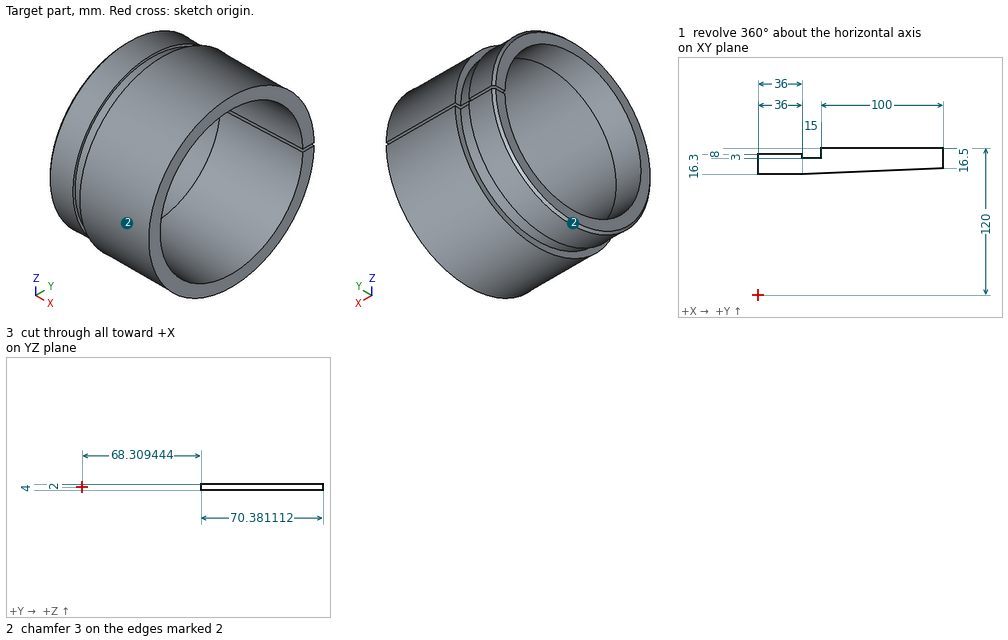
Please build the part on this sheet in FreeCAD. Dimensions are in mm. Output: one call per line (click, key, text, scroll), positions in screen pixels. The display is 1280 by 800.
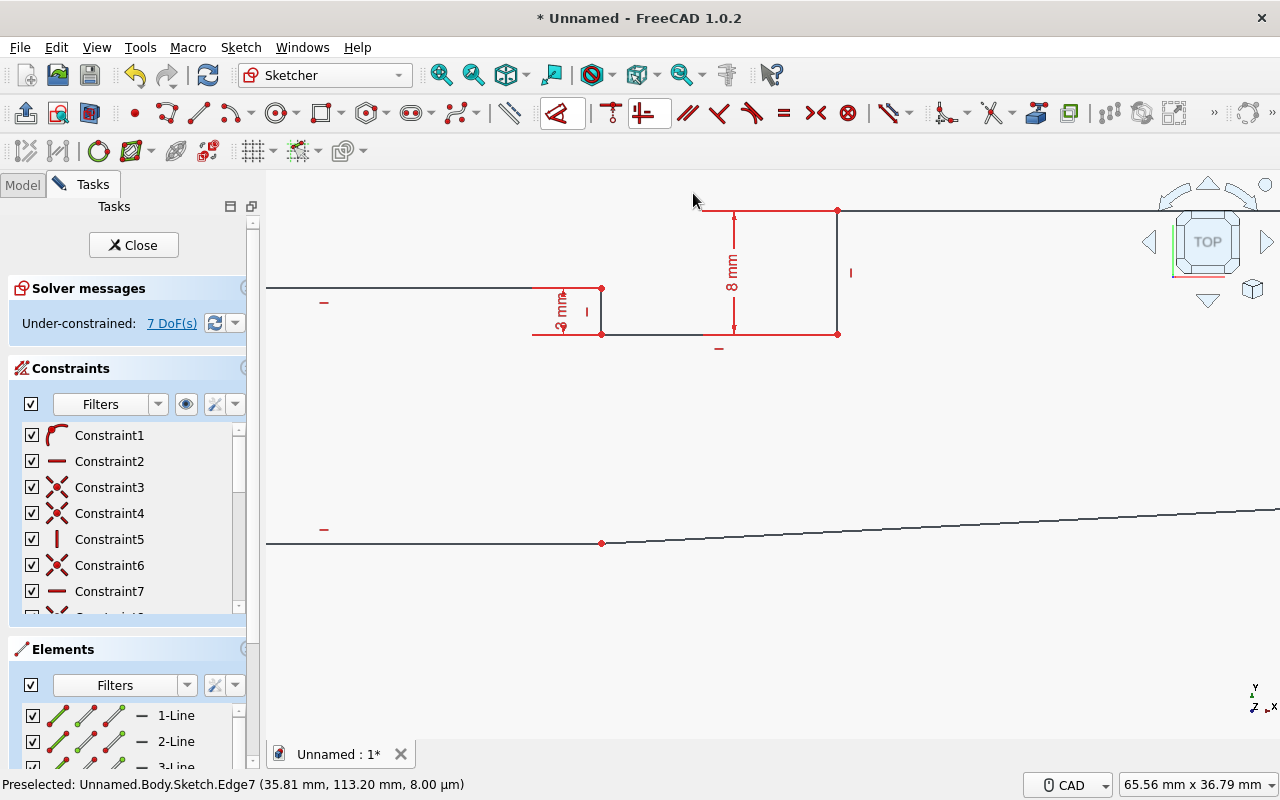
scroll(575, 282, down, 8)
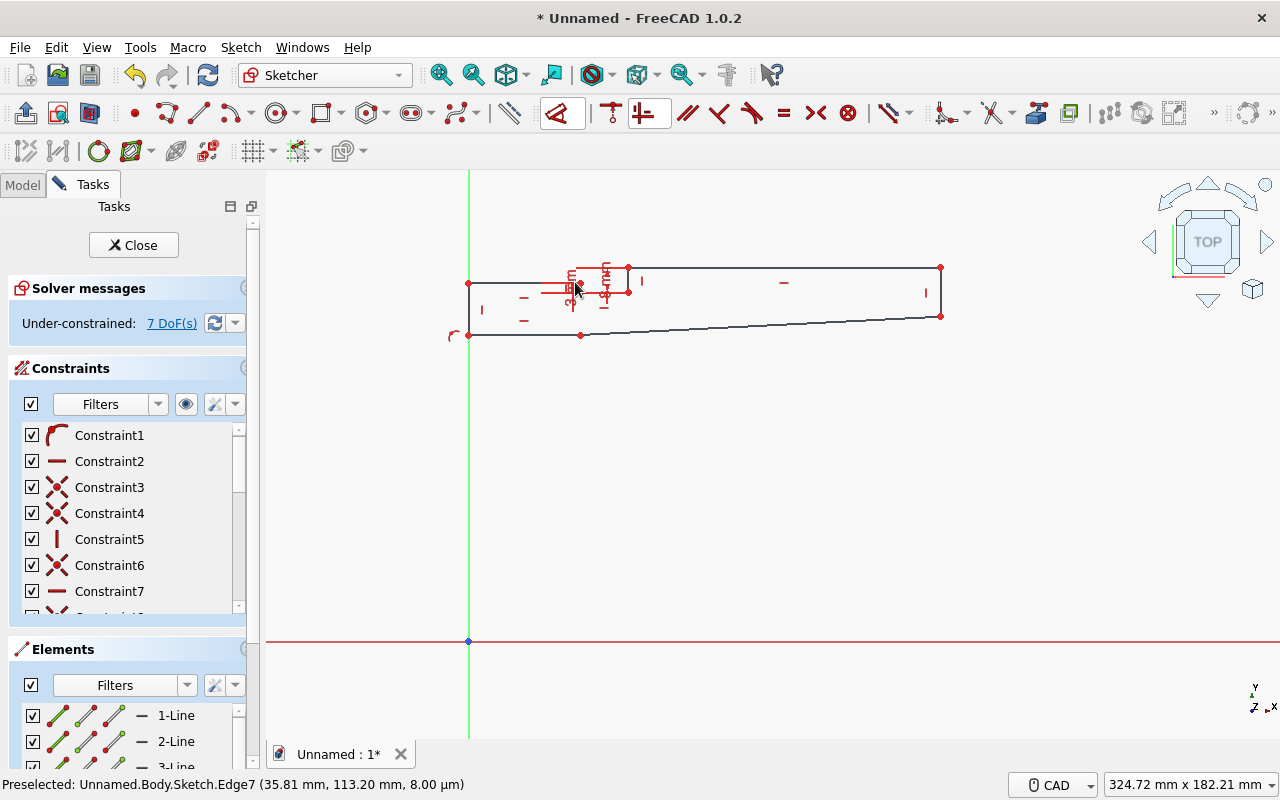
click(547, 335)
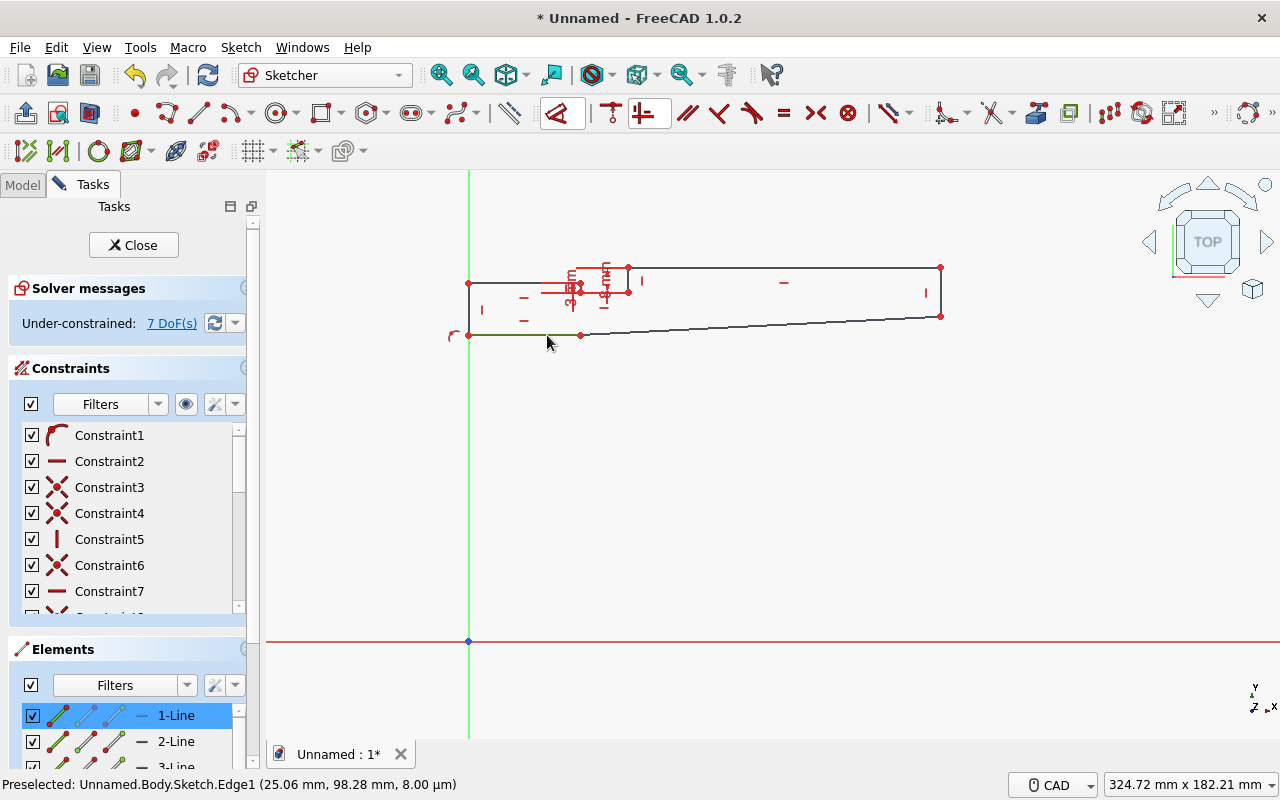
key(l)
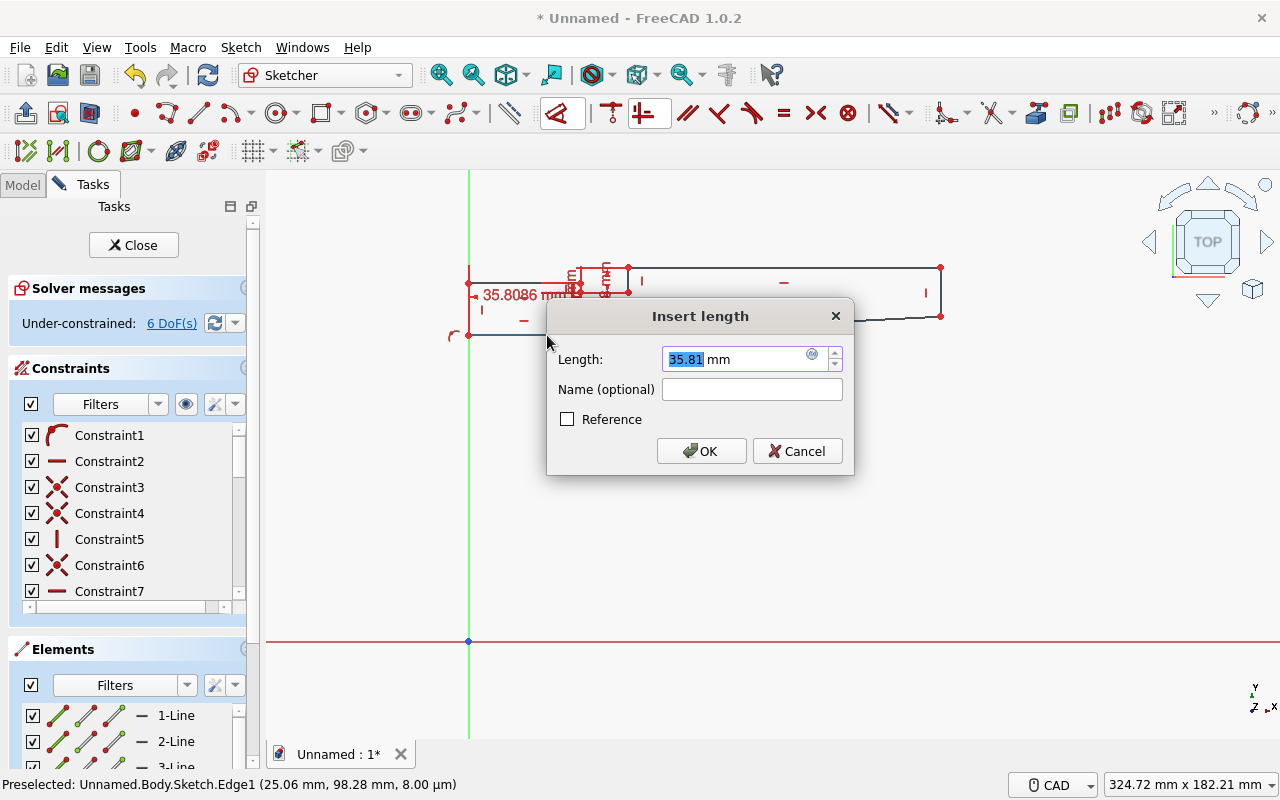
text(36)
key(Return)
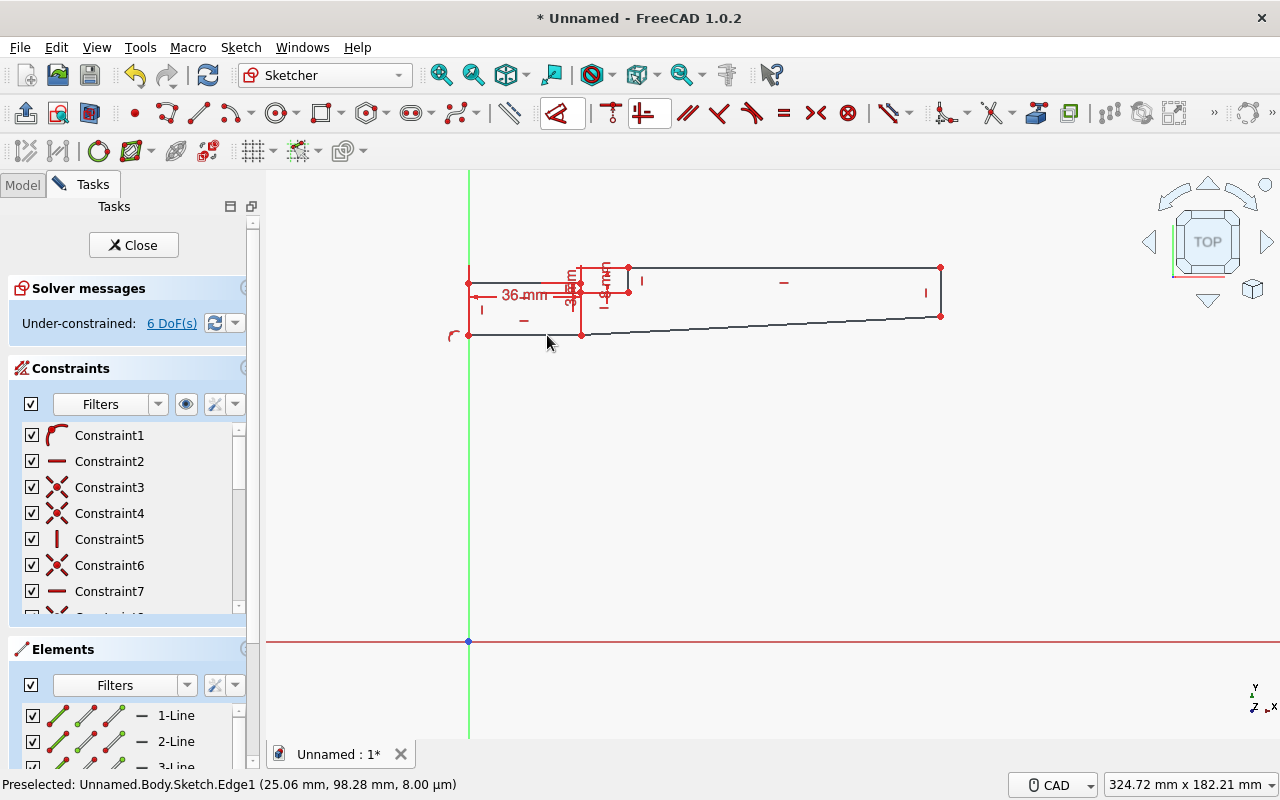
click(595, 293)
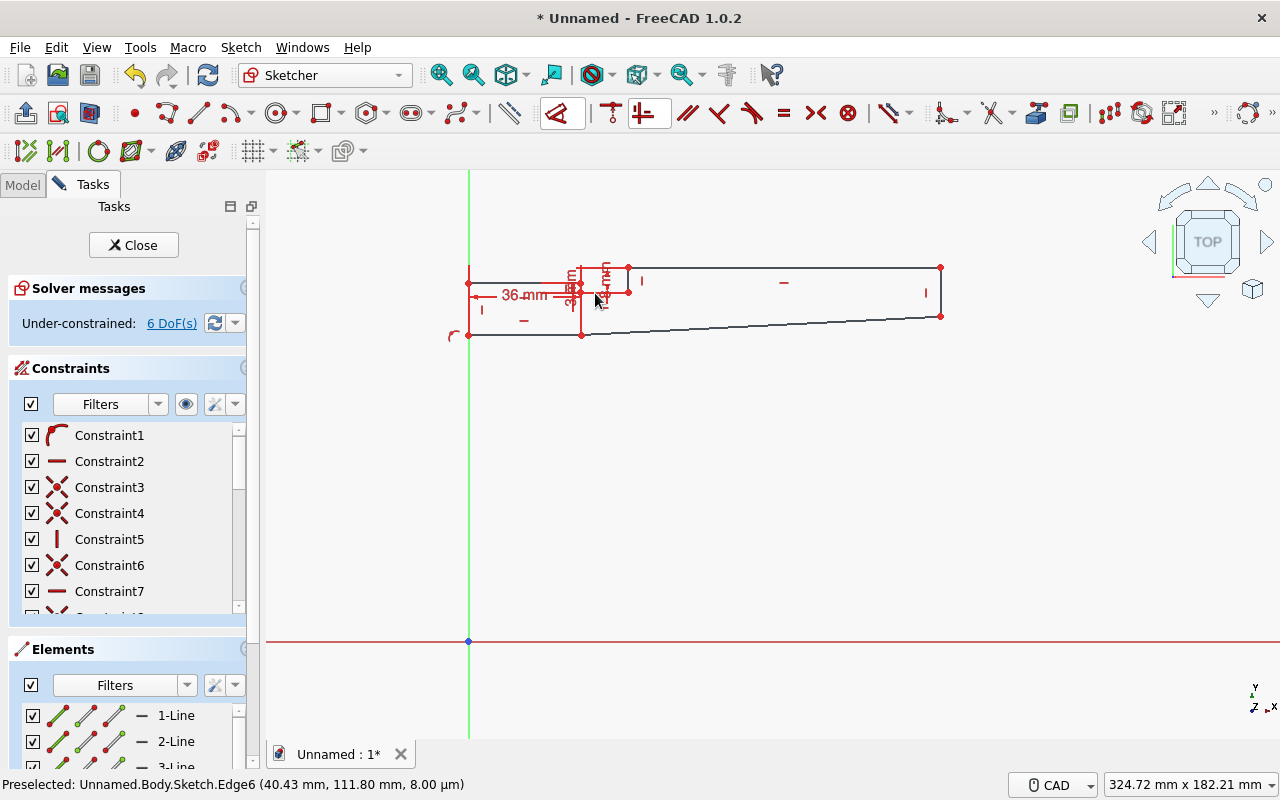
key(l)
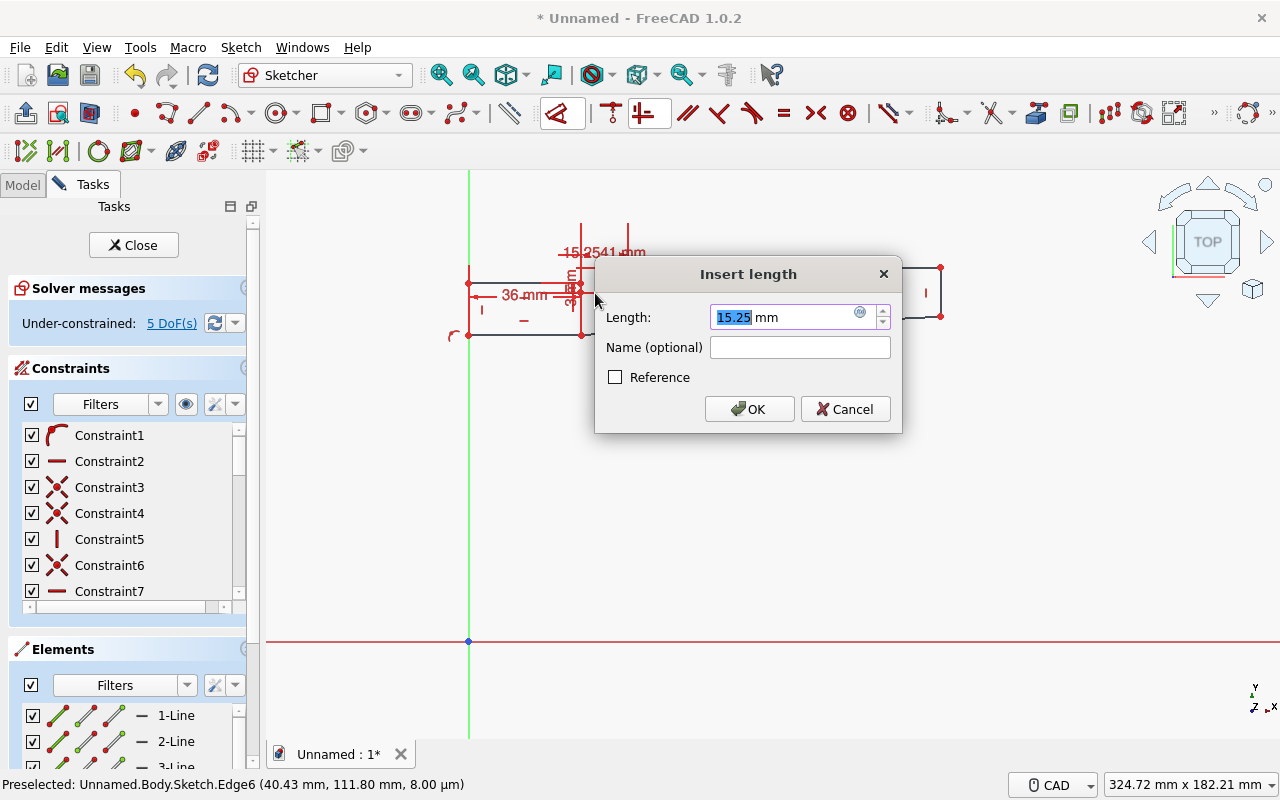
text(15)
key(Return)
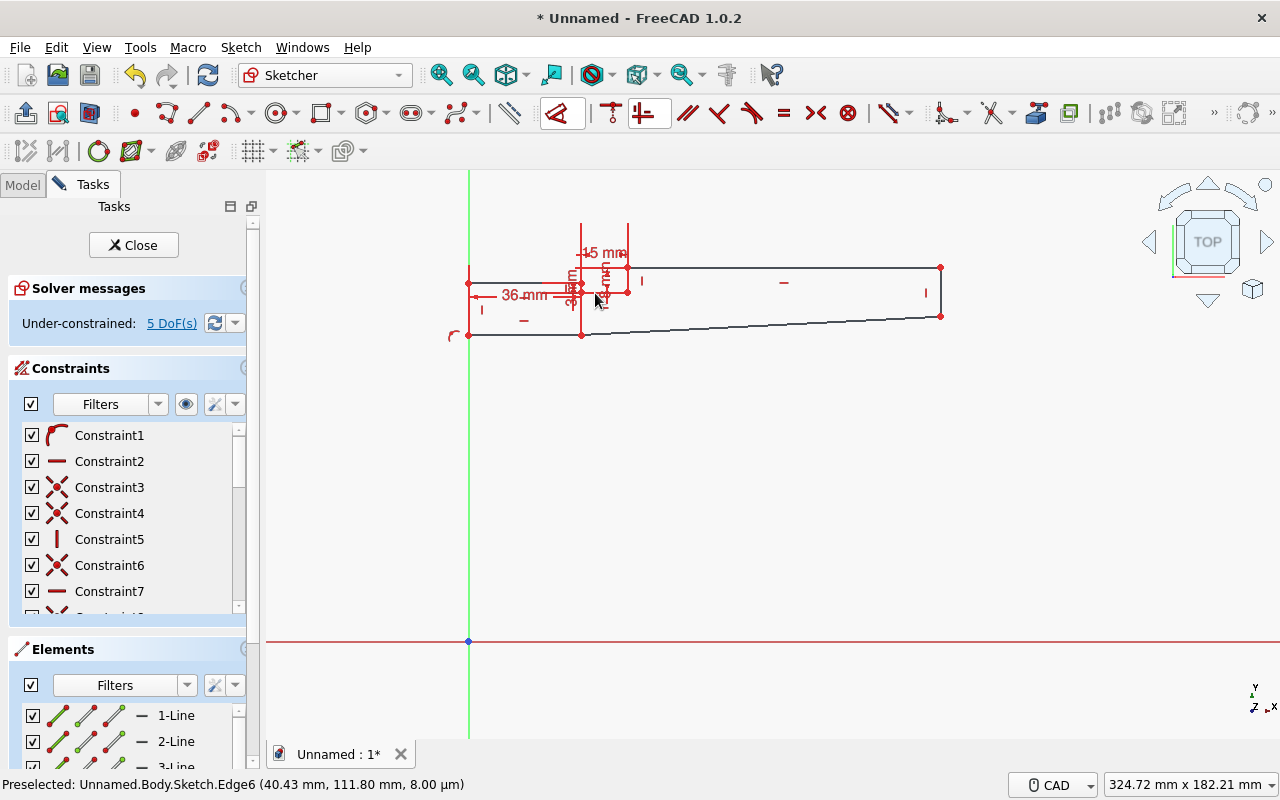
click(547, 283)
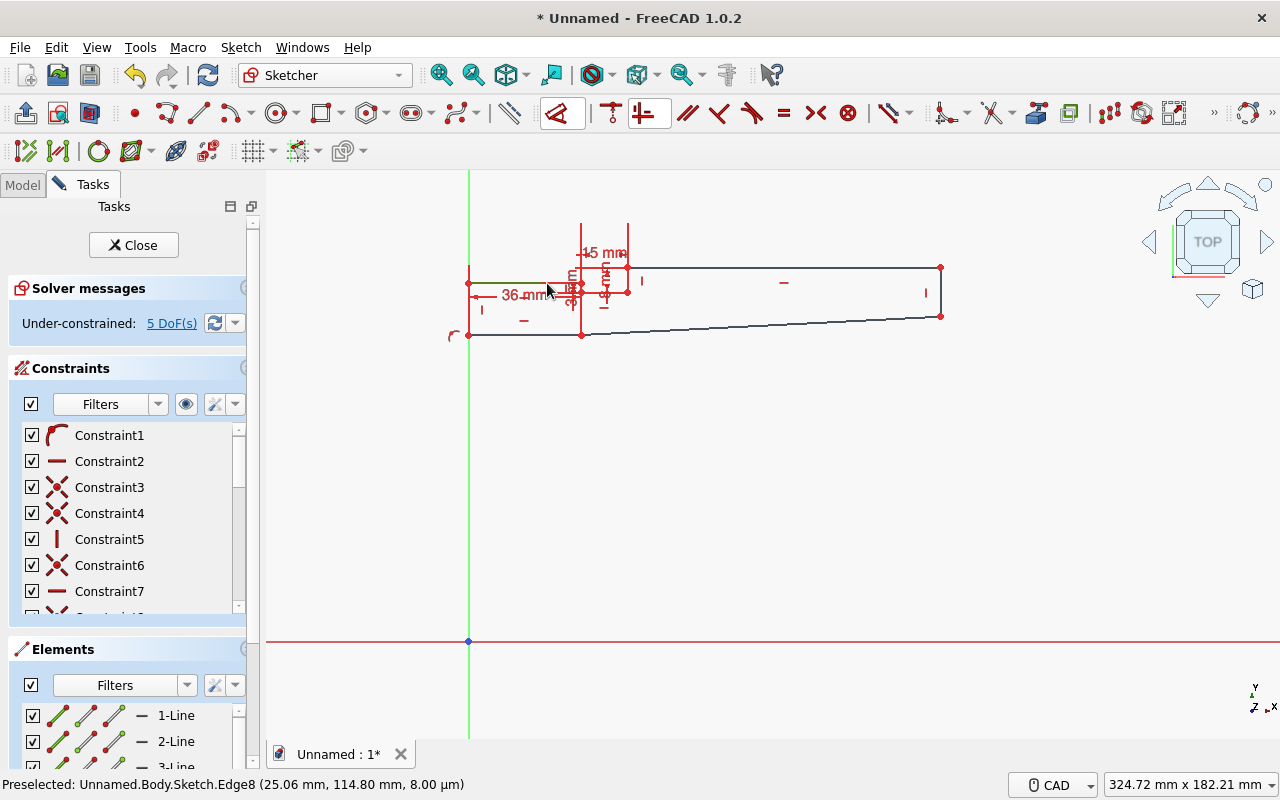
click(580, 114)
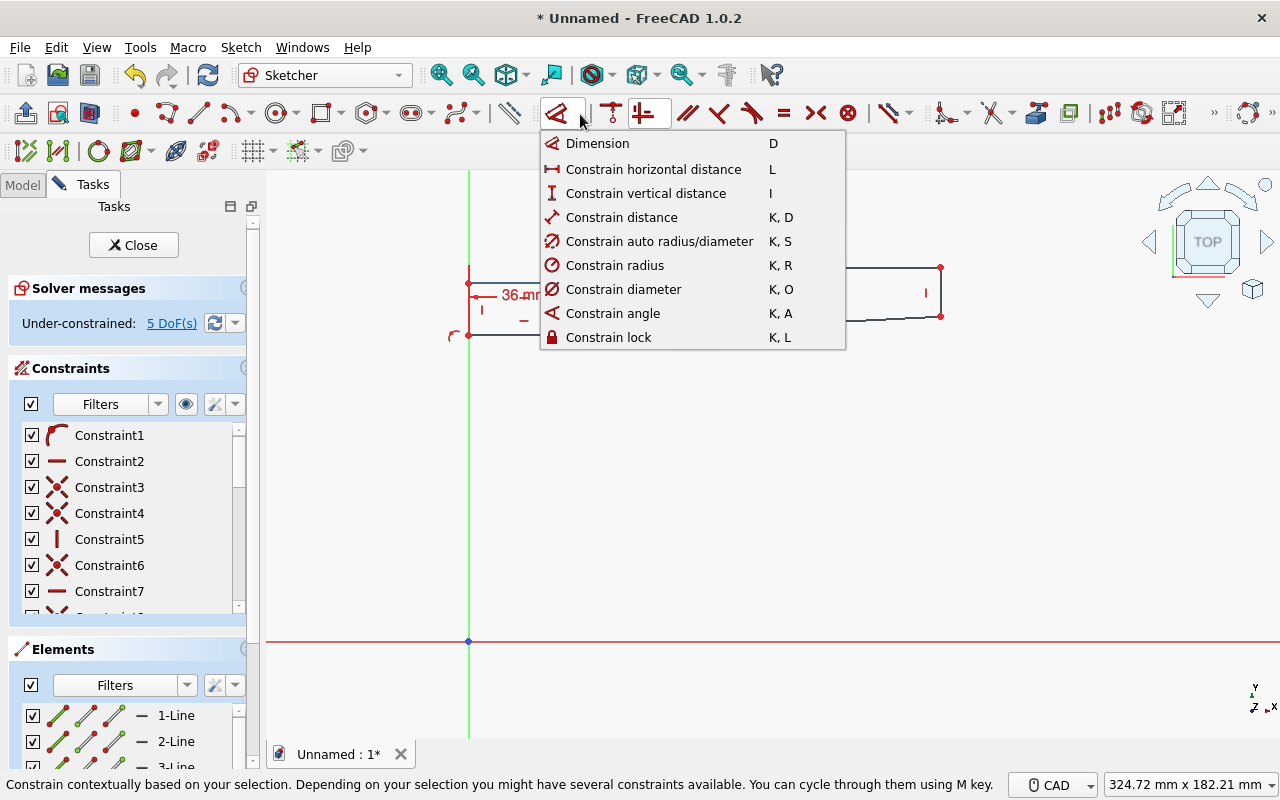
click(693, 169)